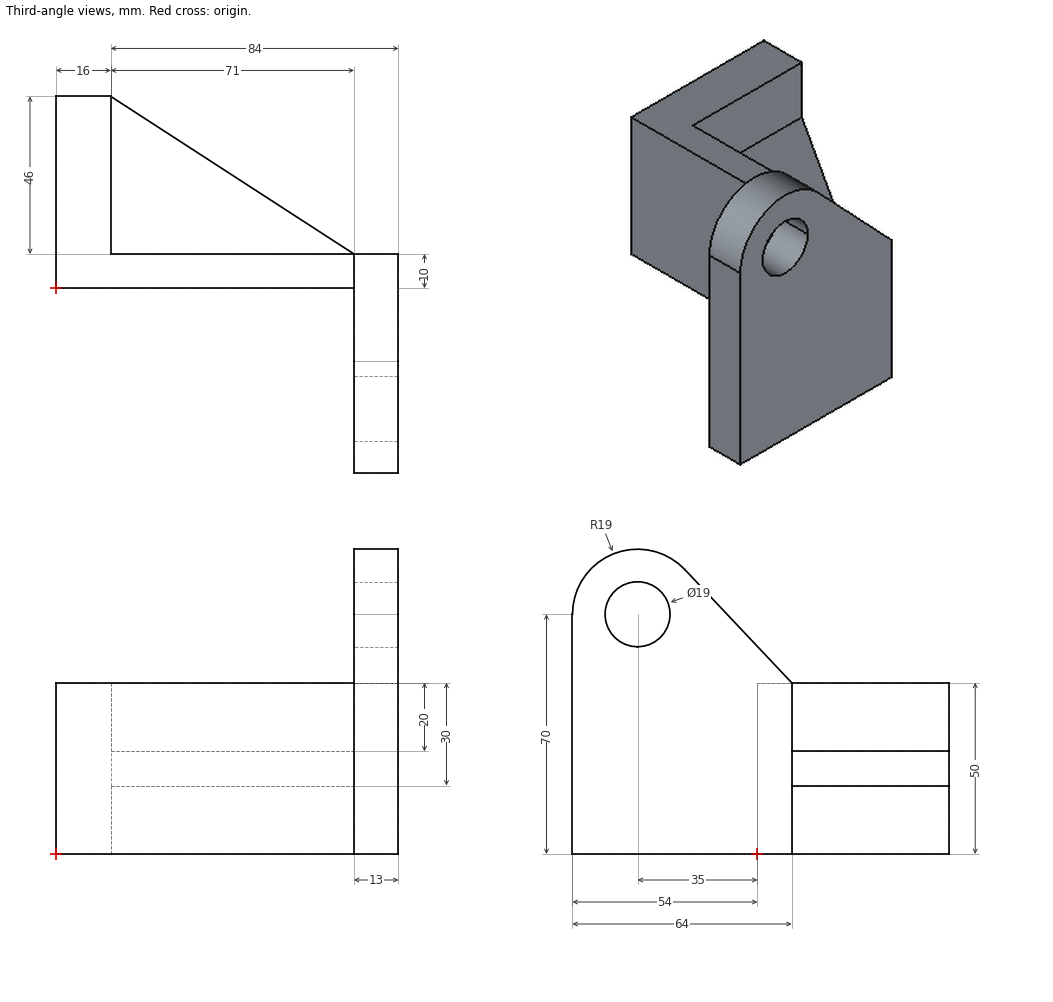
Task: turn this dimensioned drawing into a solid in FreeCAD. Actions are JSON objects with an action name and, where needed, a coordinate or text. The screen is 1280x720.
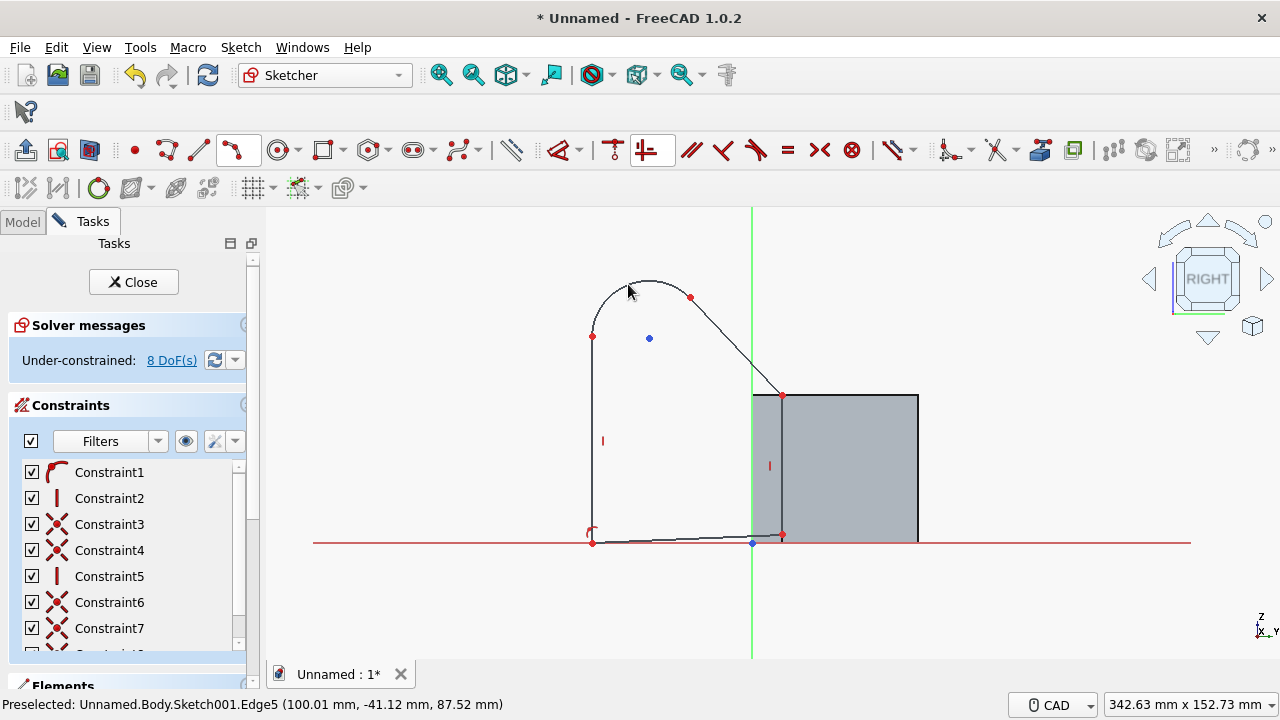
{"action": "left_click", "coordinate": [592, 399]}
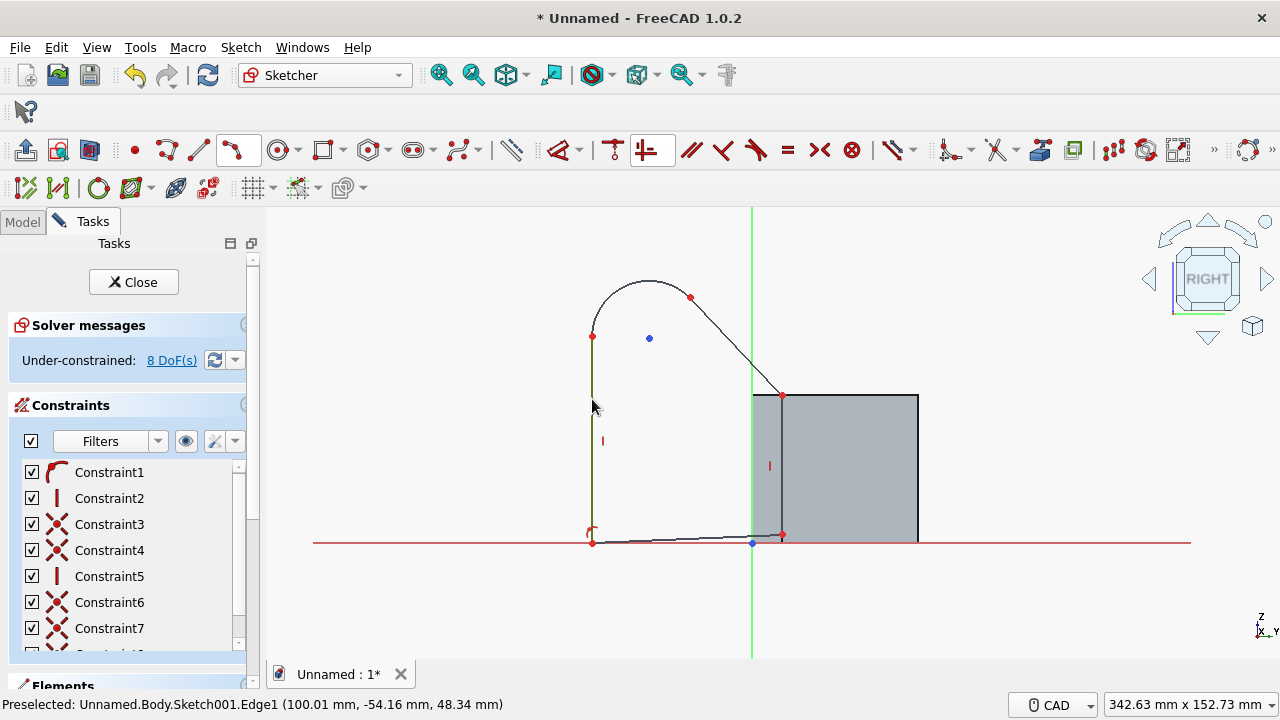
{"action": "left_click", "coordinate": [654, 281]}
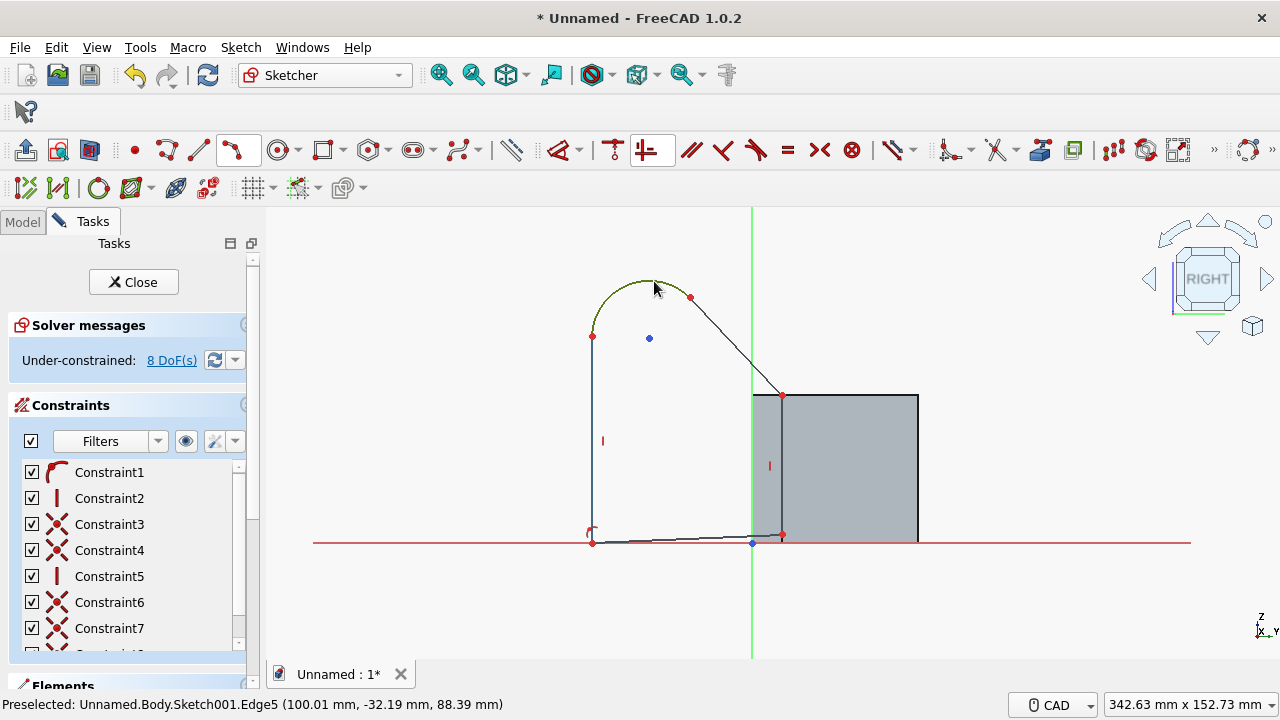
{"action": "left_click", "coordinate": [756, 150]}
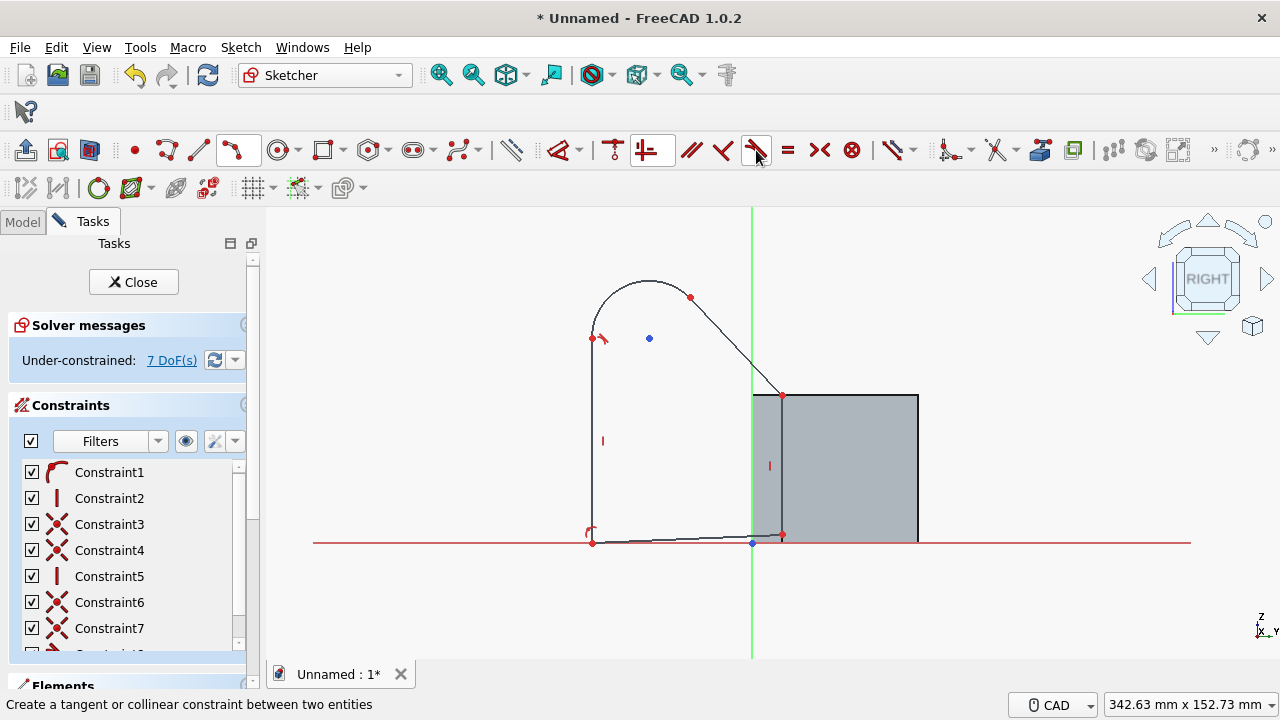
{"action": "left_click", "coordinate": [754, 367]}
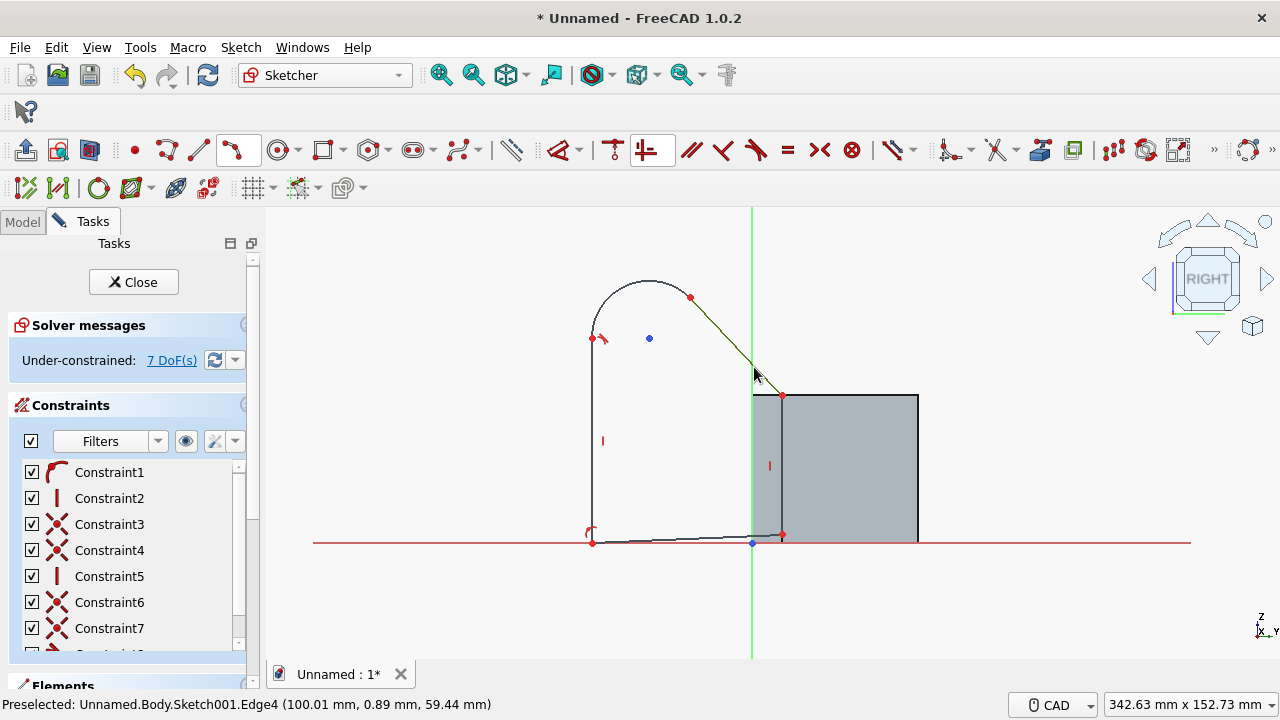
{"action": "left_click", "coordinate": [654, 281]}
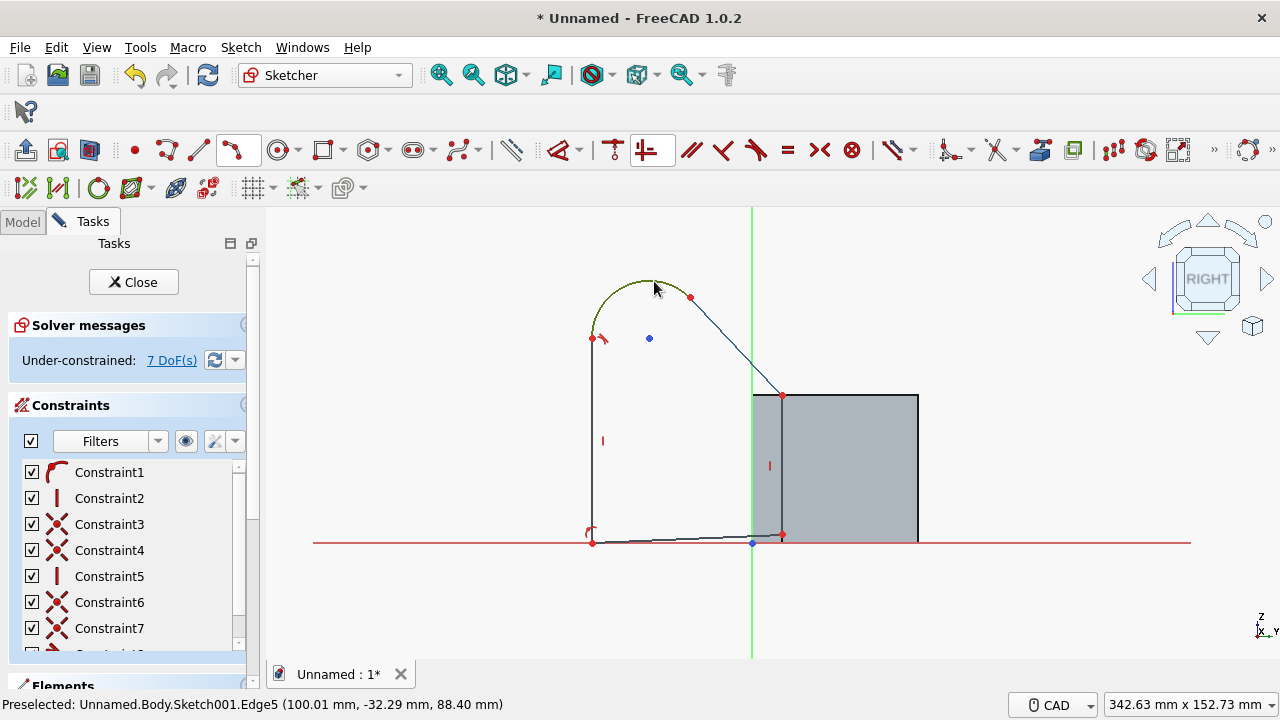
{"action": "key", "text": "t"}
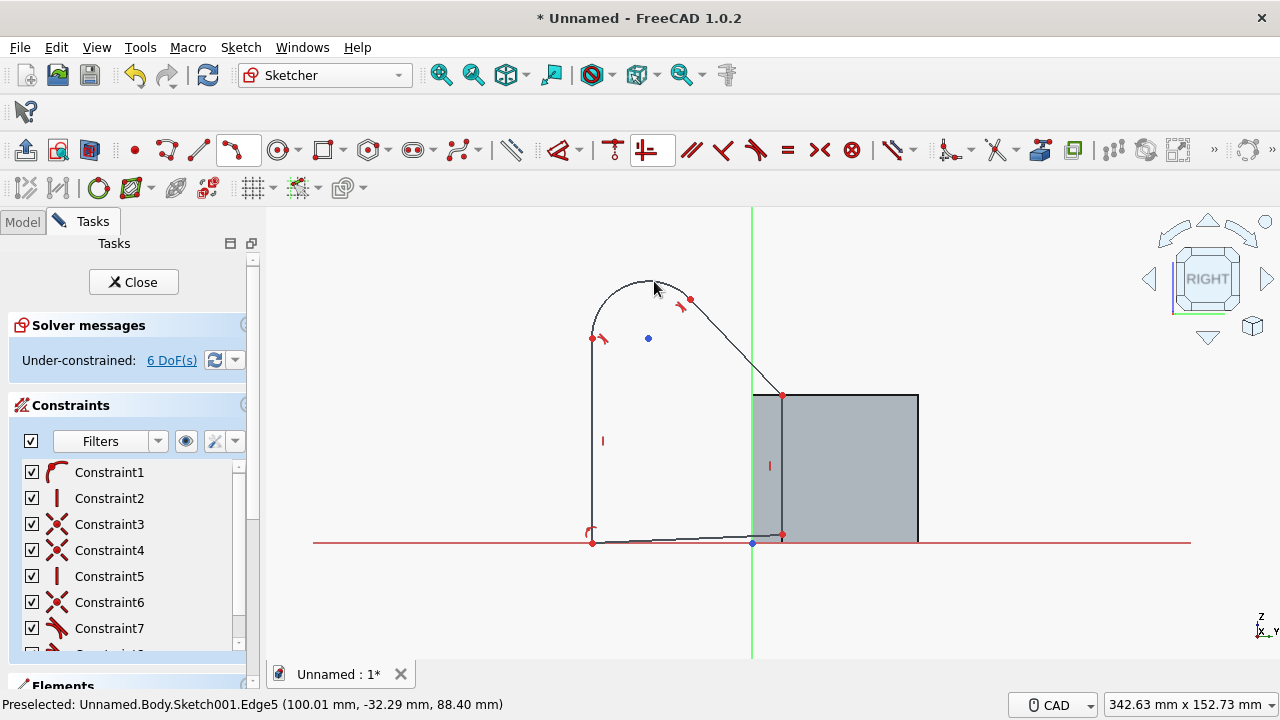
{"action": "left_click", "coordinate": [649, 541]}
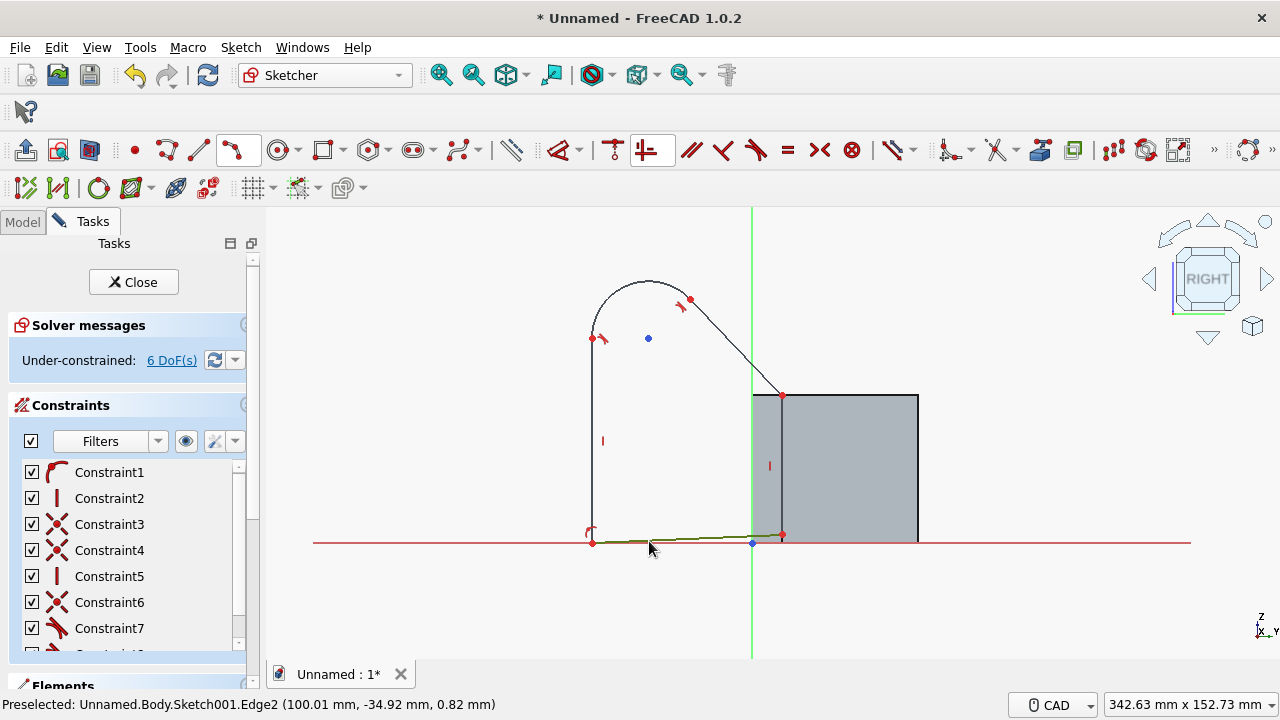
{"action": "key", "text": "h"}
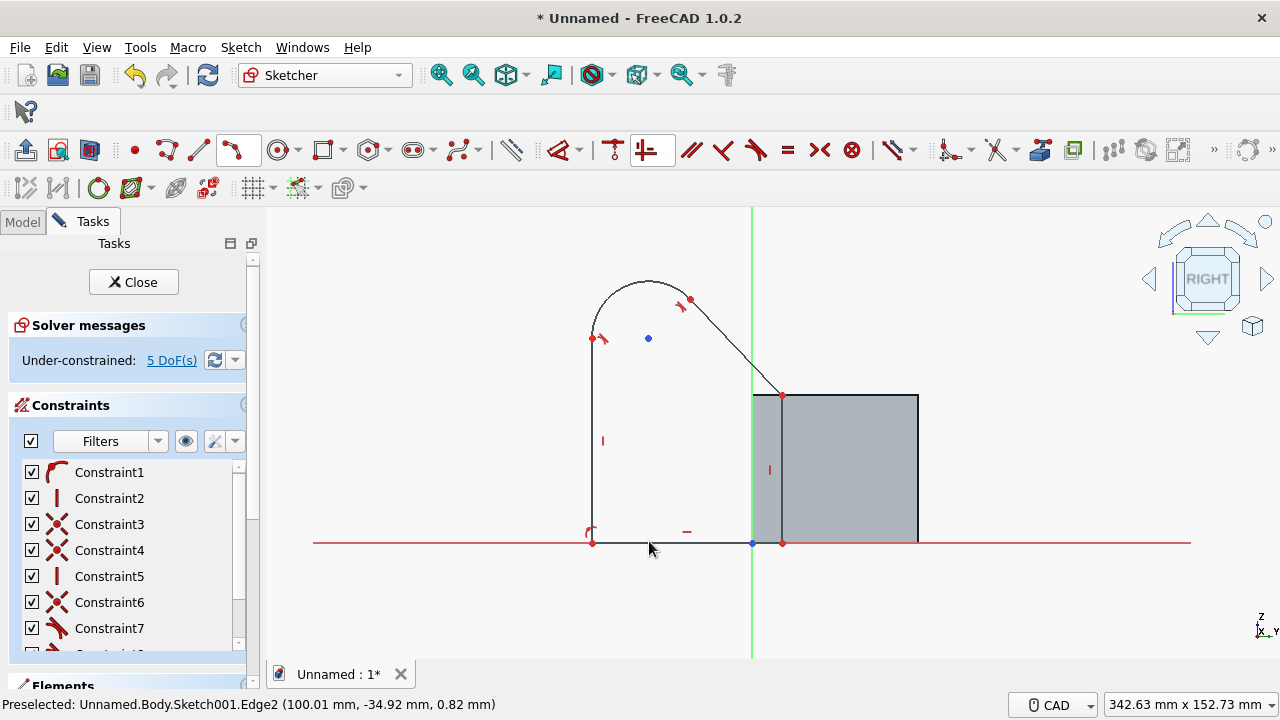
{"action": "key", "text": "d"}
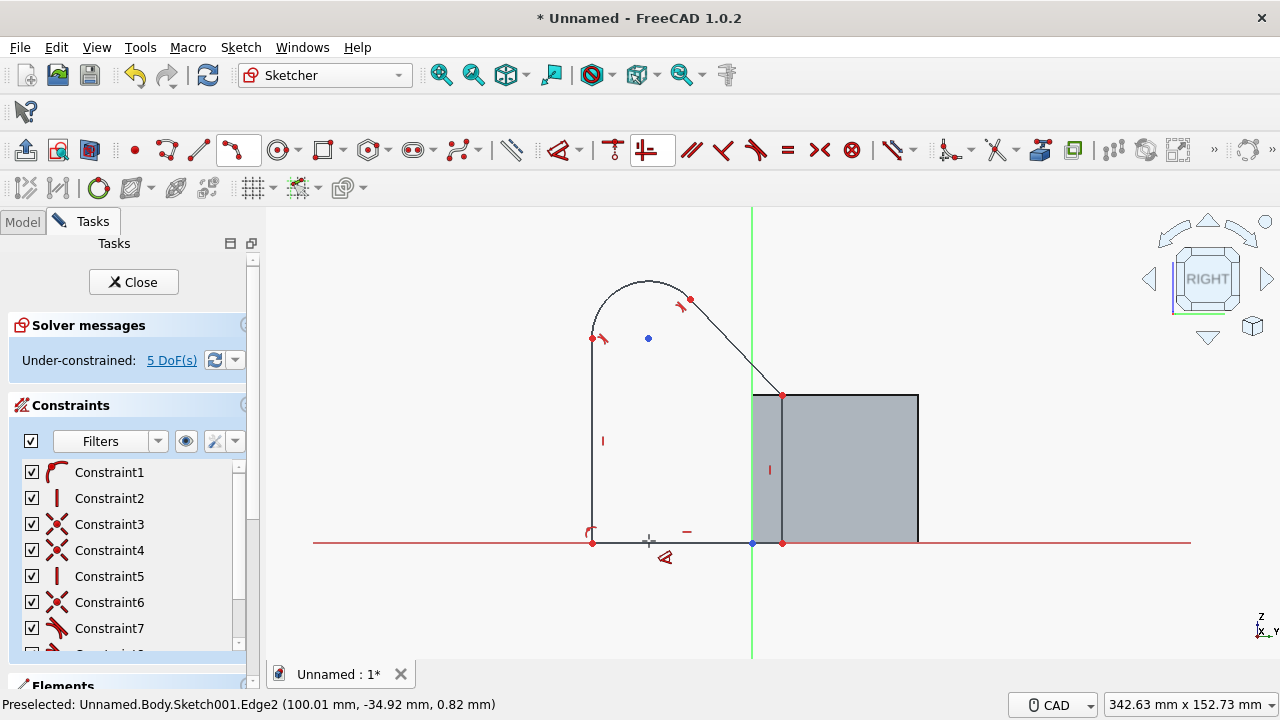
{"action": "left_click", "coordinate": [654, 282]}
{"action": "left_click", "coordinate": [657, 250]}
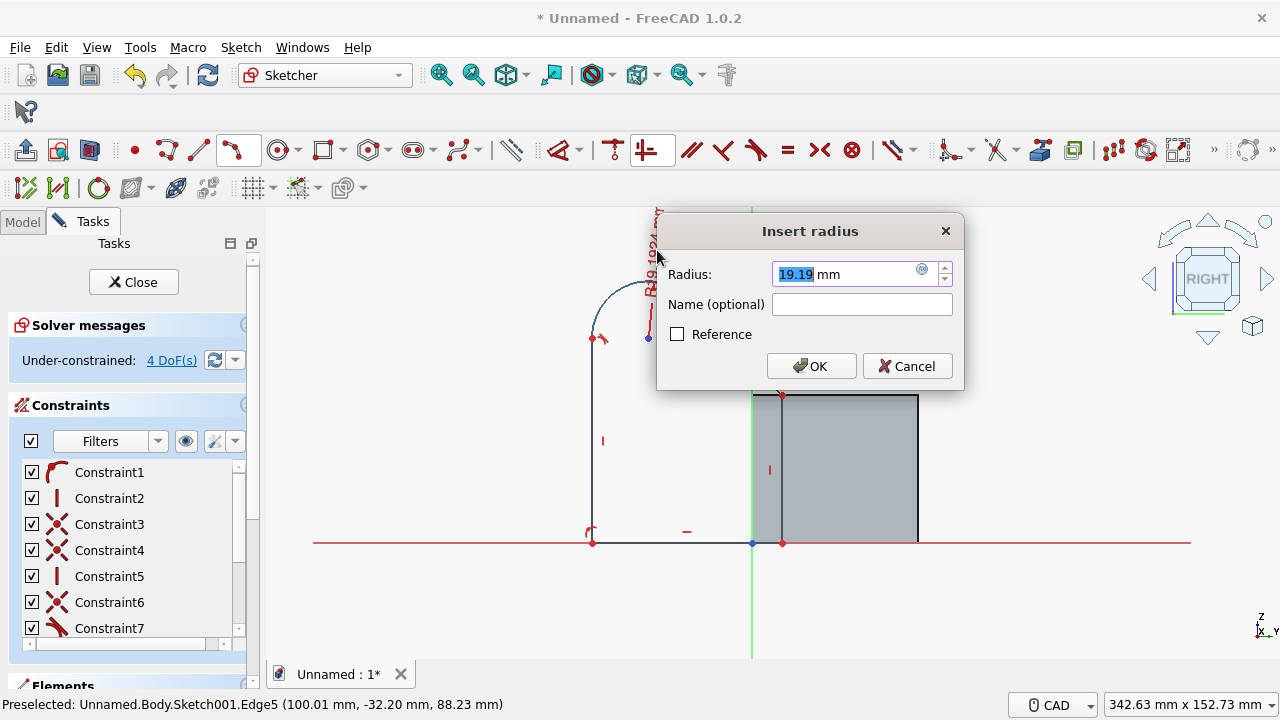
{"action": "type", "text": "19"}
{"action": "key", "text": "Return"}